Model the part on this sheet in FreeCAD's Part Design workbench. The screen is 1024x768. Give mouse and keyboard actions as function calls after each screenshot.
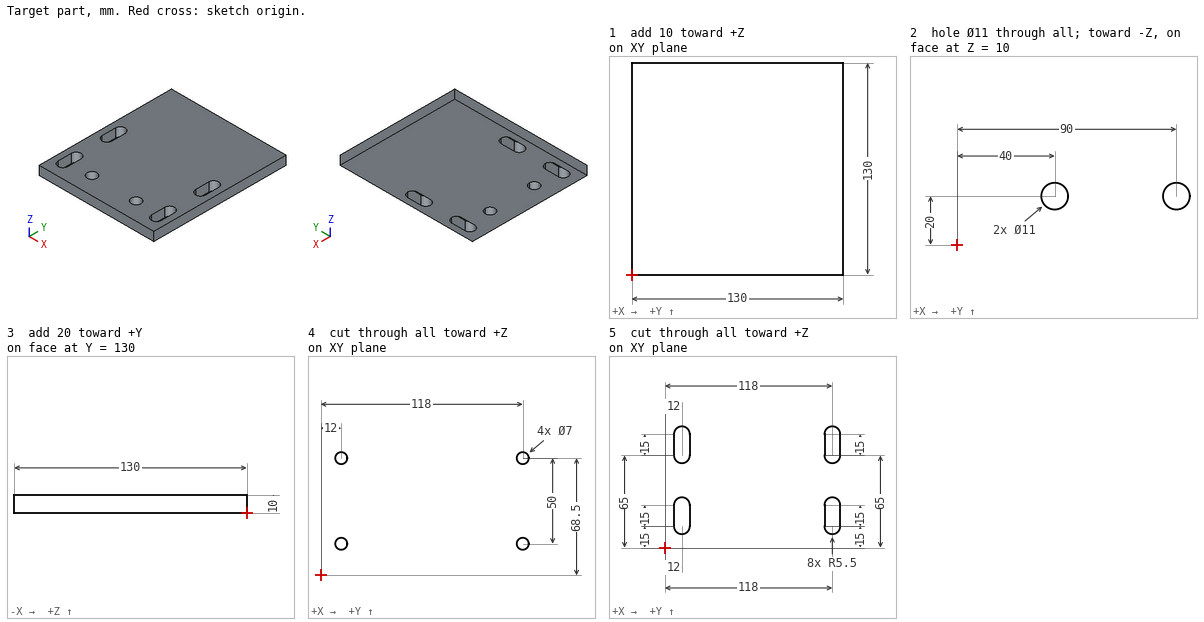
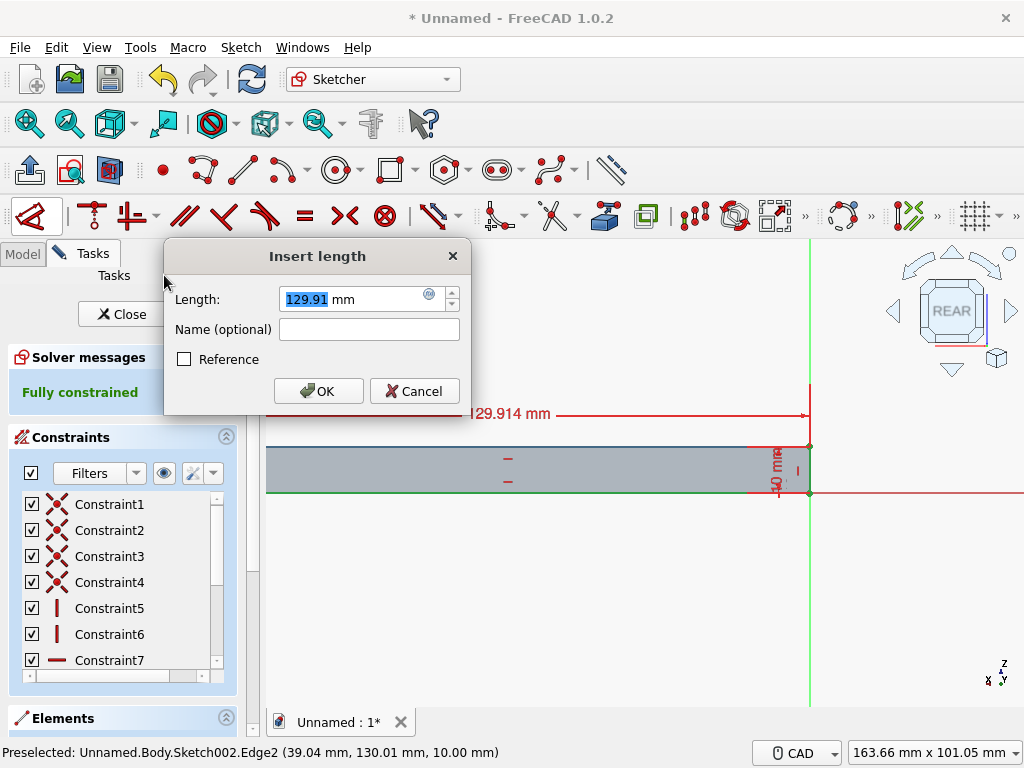
text(130)
key(Return)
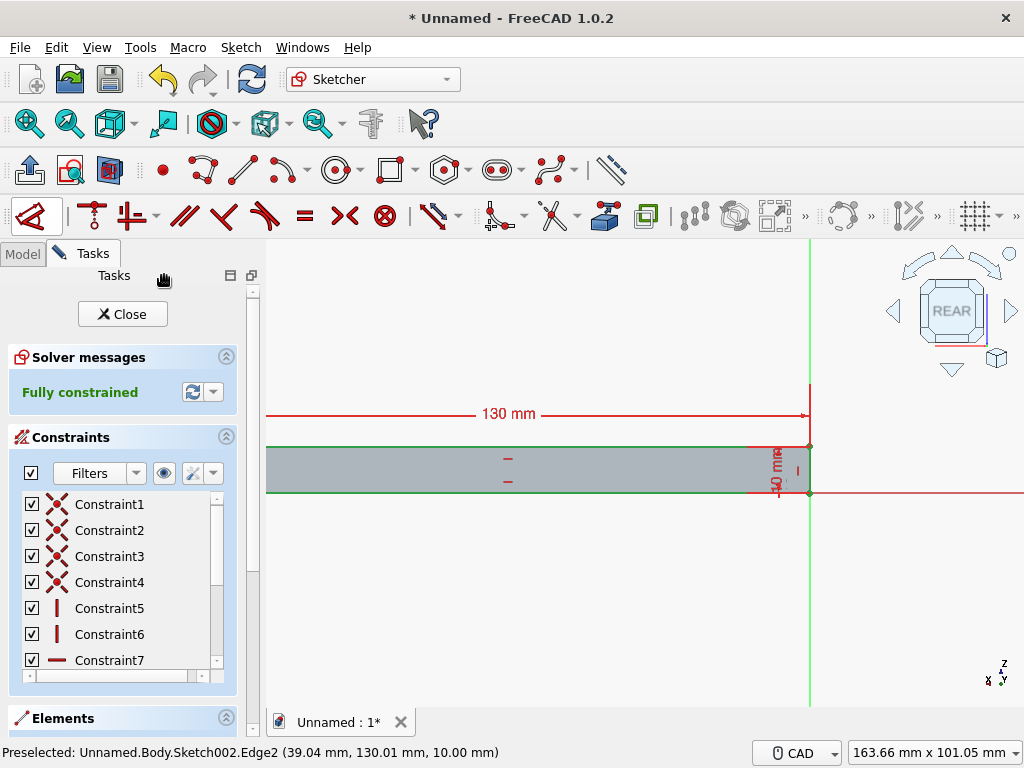
click(123, 314)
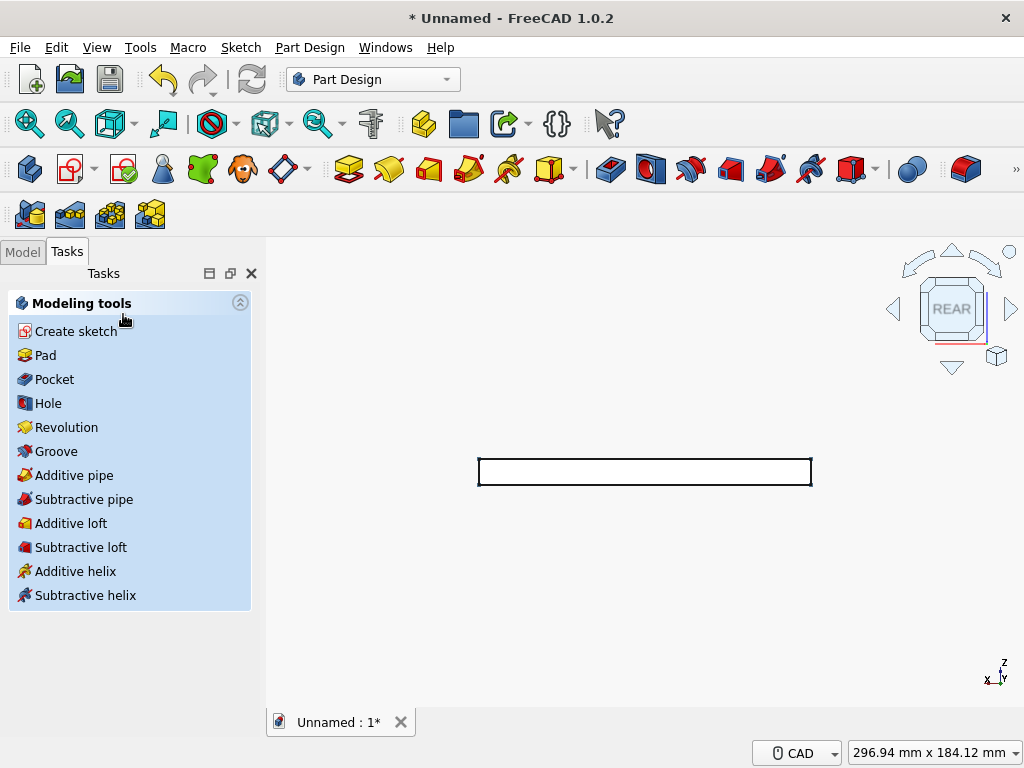
click(350, 170)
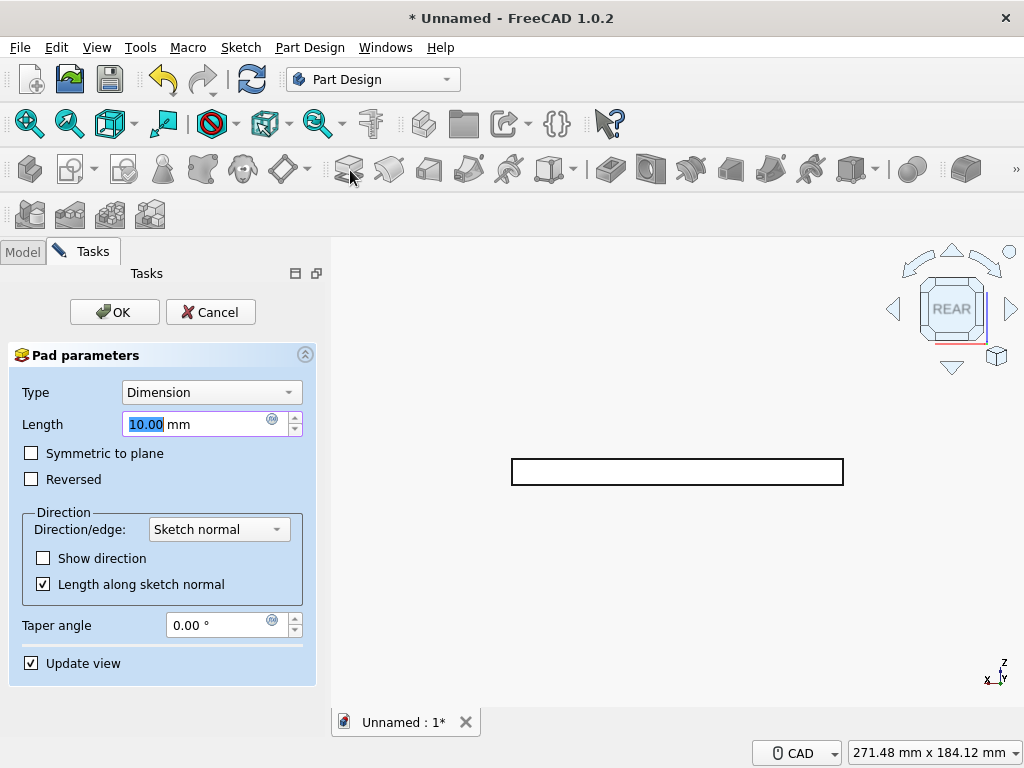
text(20)
key(Tab)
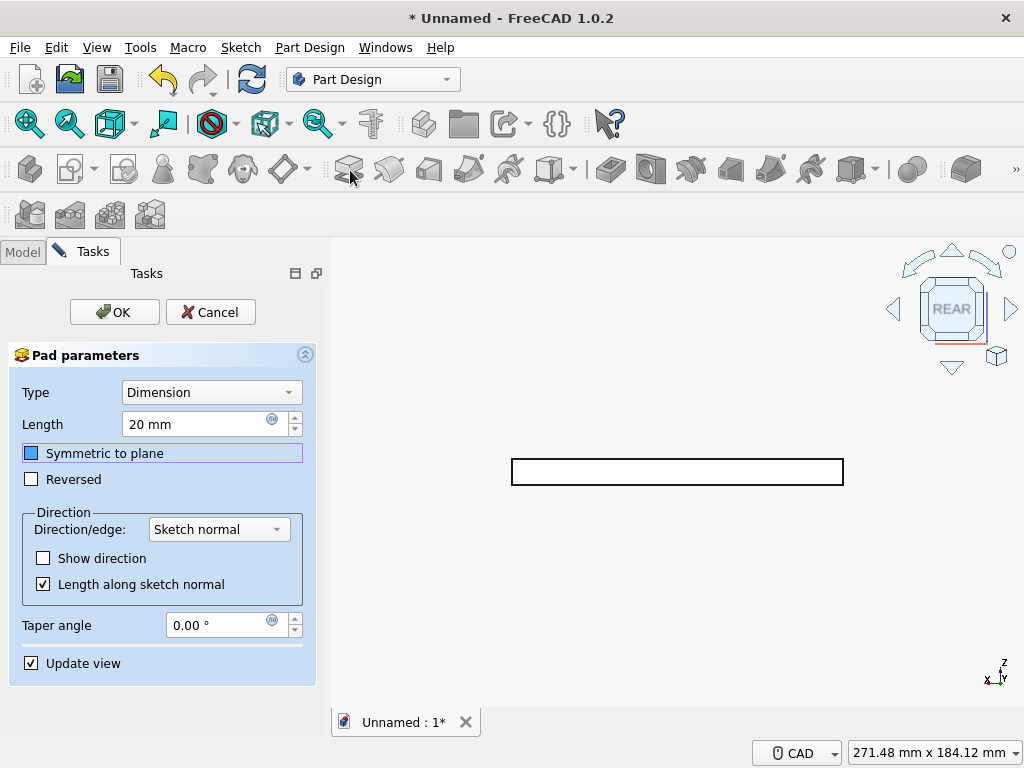
click(115, 312)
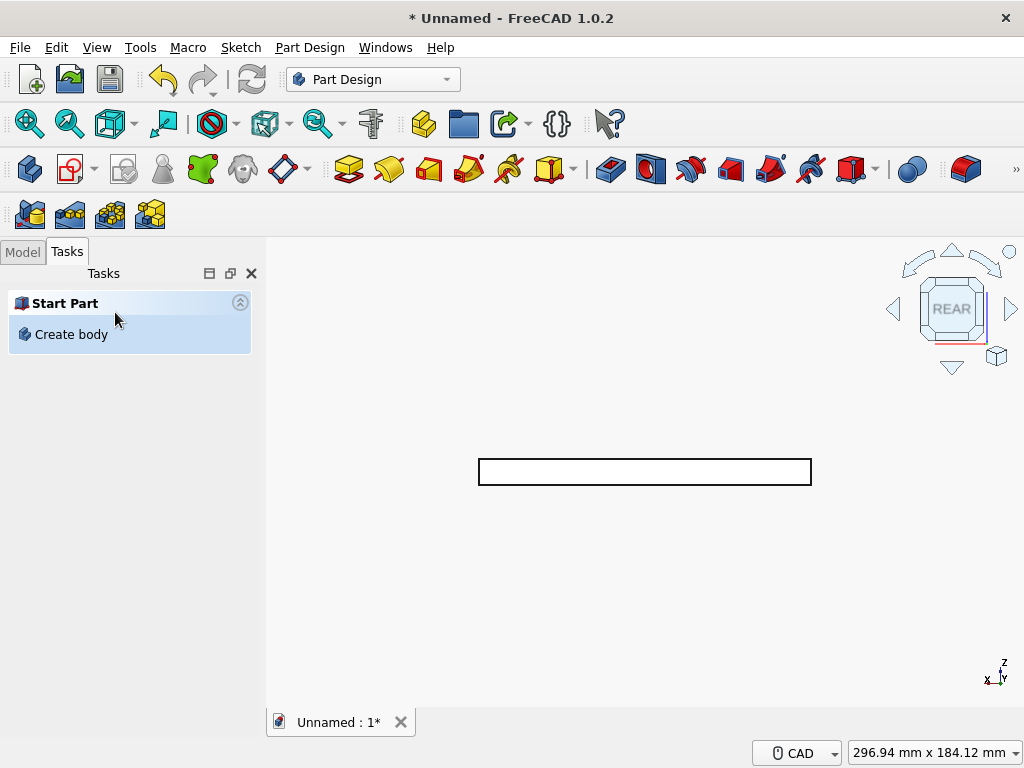
click(30, 124)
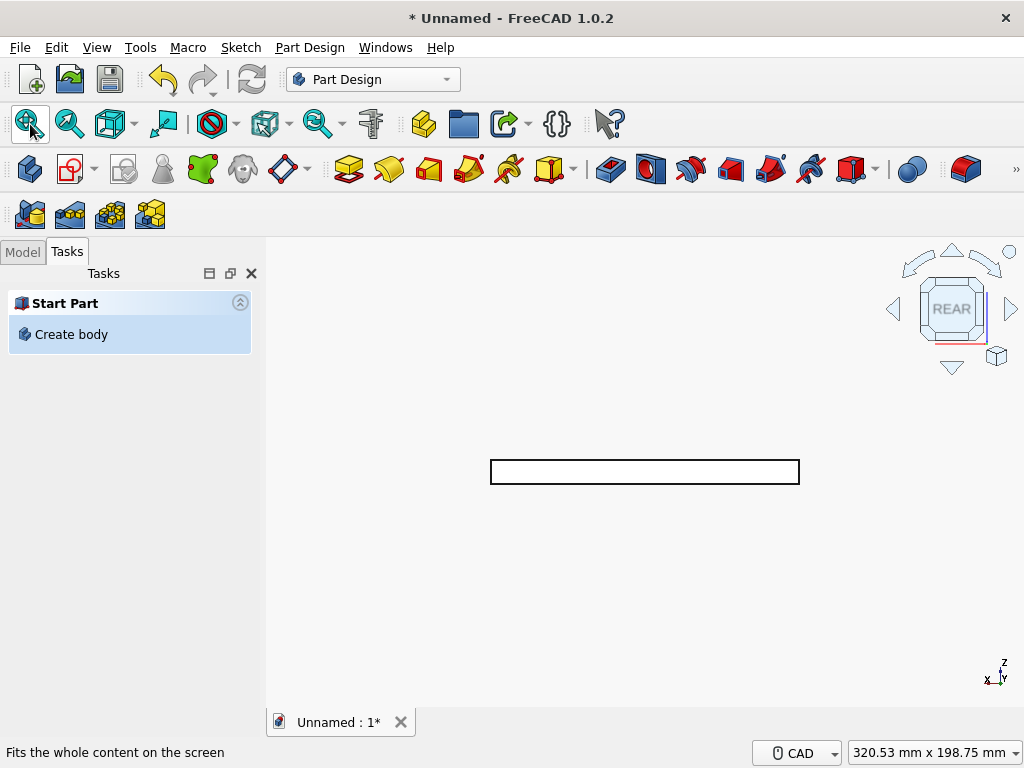
click(70, 170)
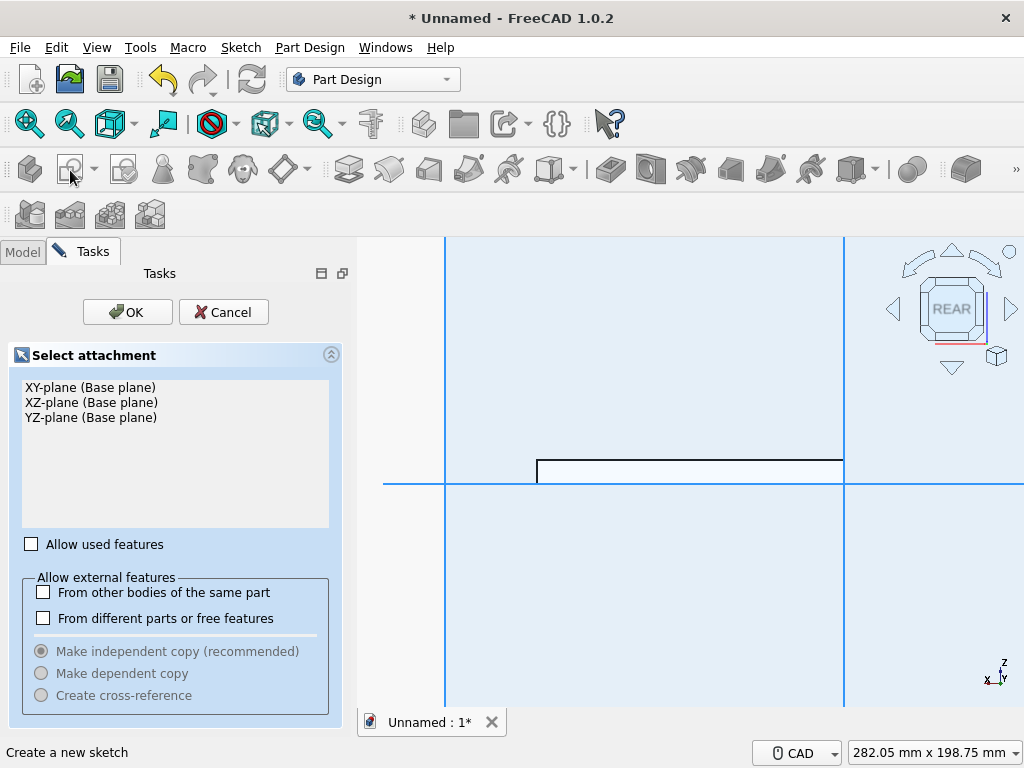
click(82, 388)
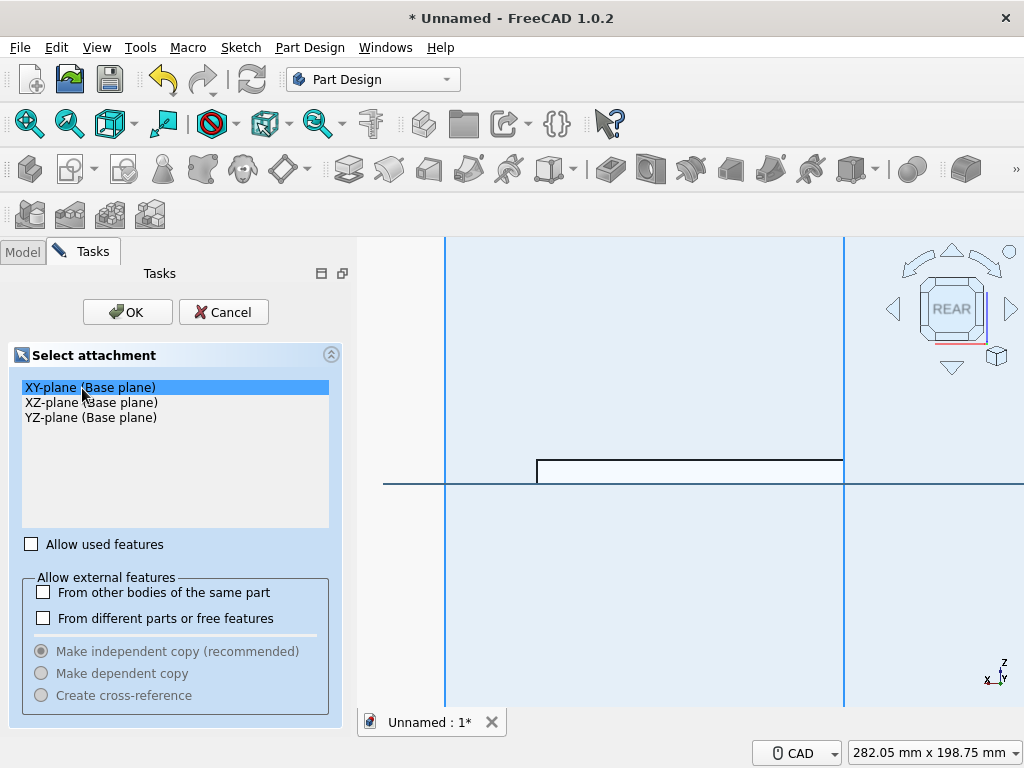
click(128, 312)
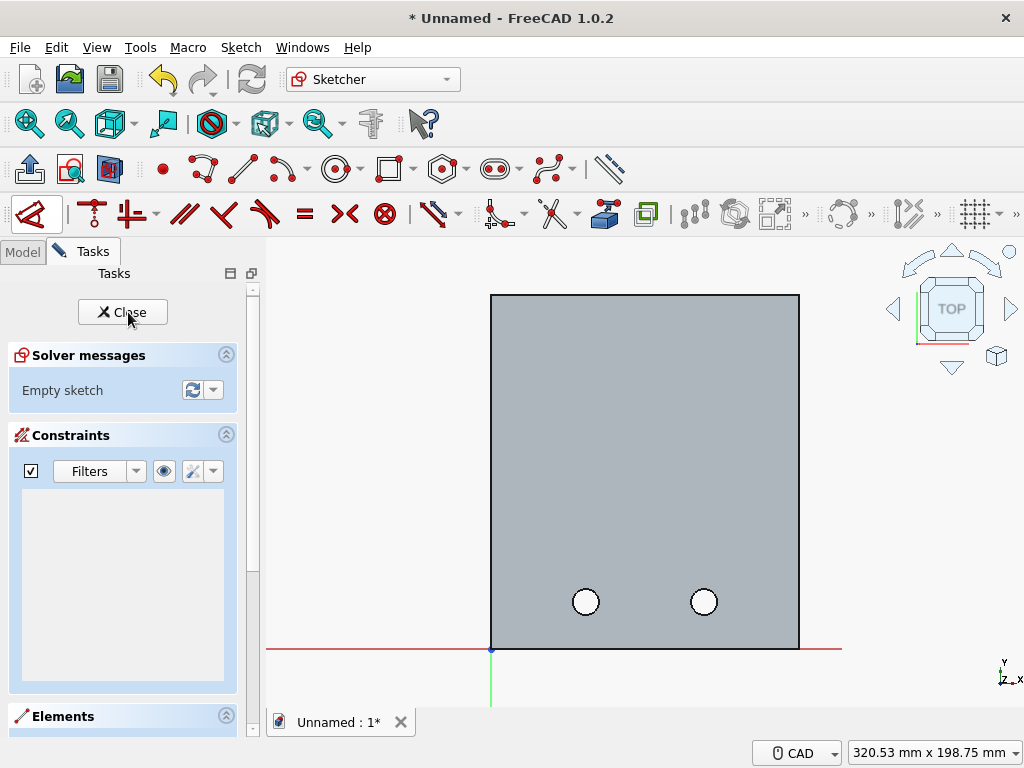
click(110, 170)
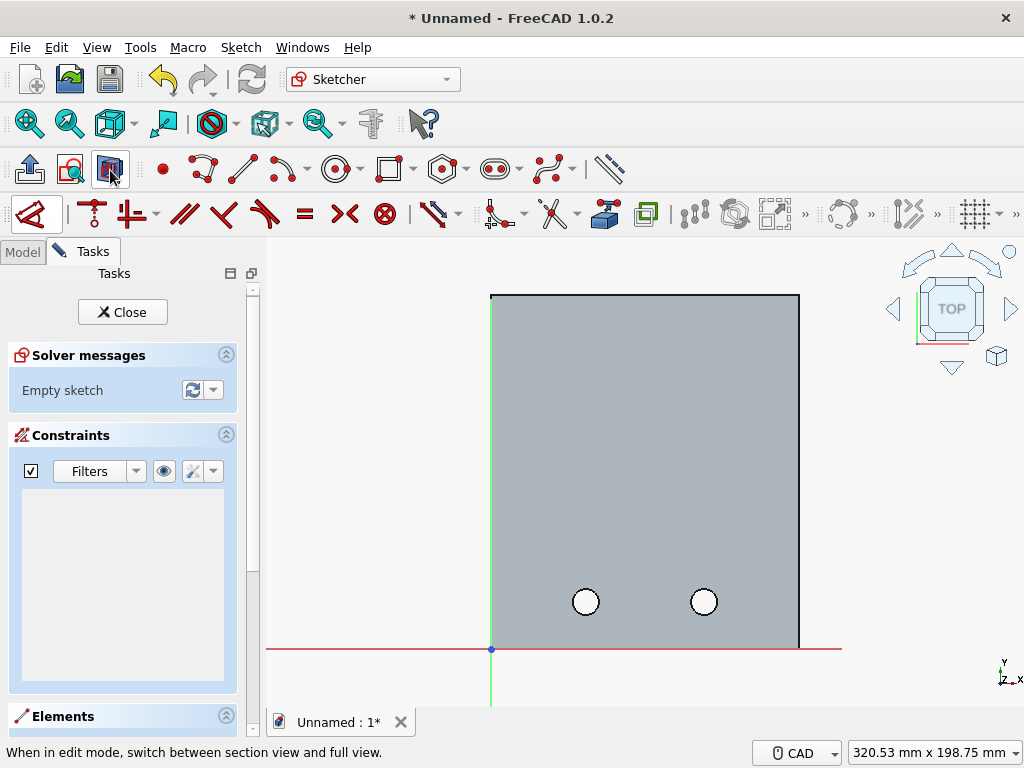
scroll(754, 679, up, 2)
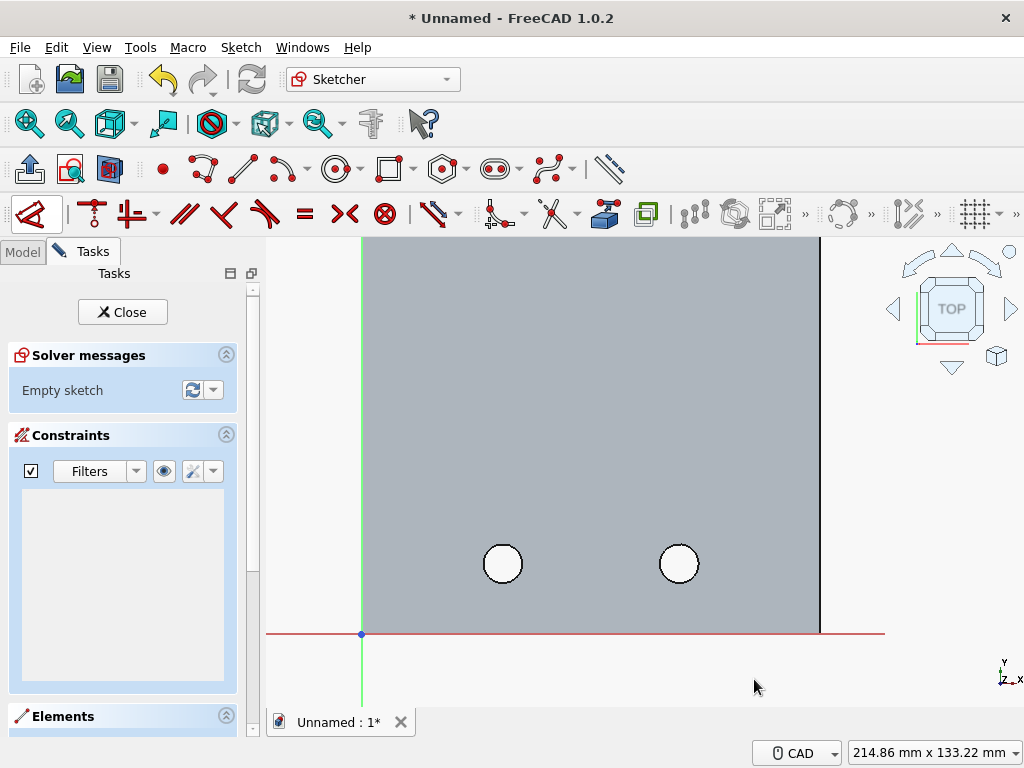
click(336, 170)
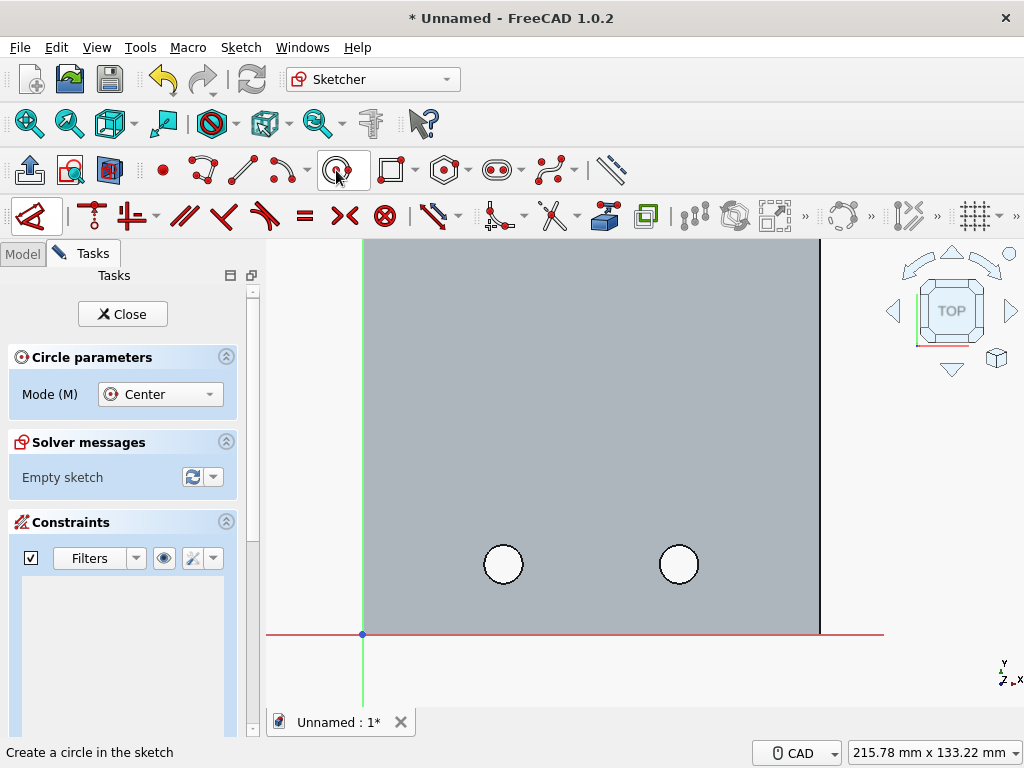
scroll(777, 394, up, 4)